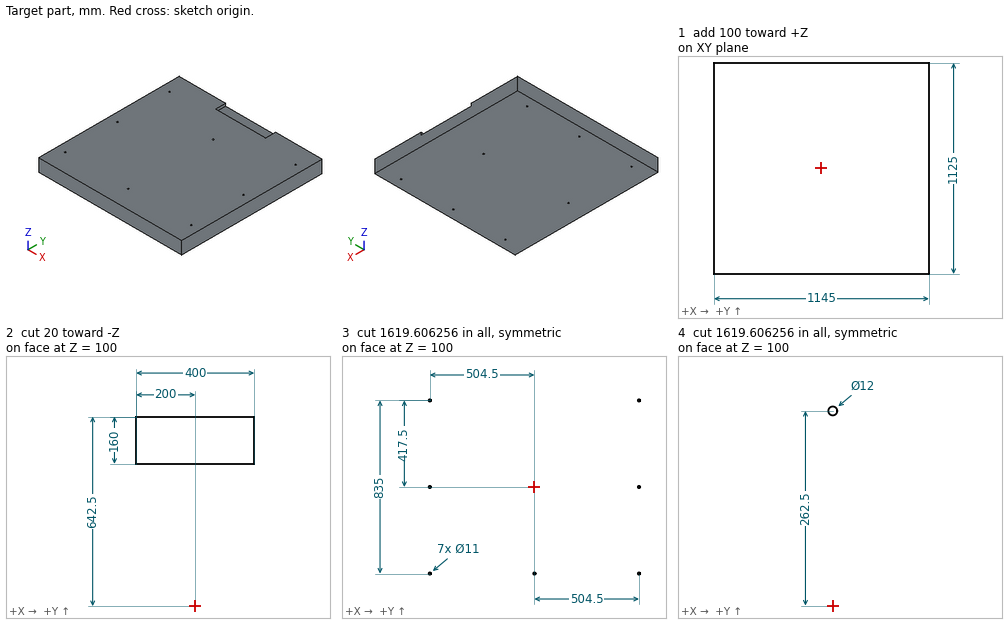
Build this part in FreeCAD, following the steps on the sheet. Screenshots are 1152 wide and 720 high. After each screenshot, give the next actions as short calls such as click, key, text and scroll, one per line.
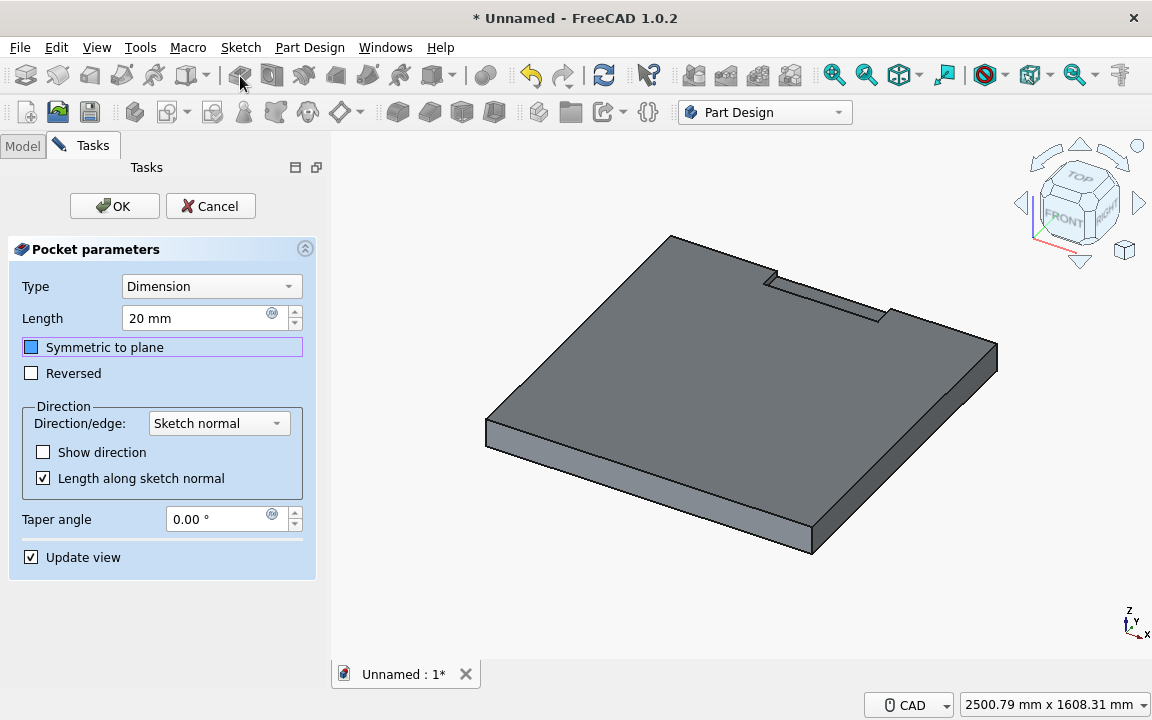
click(115, 206)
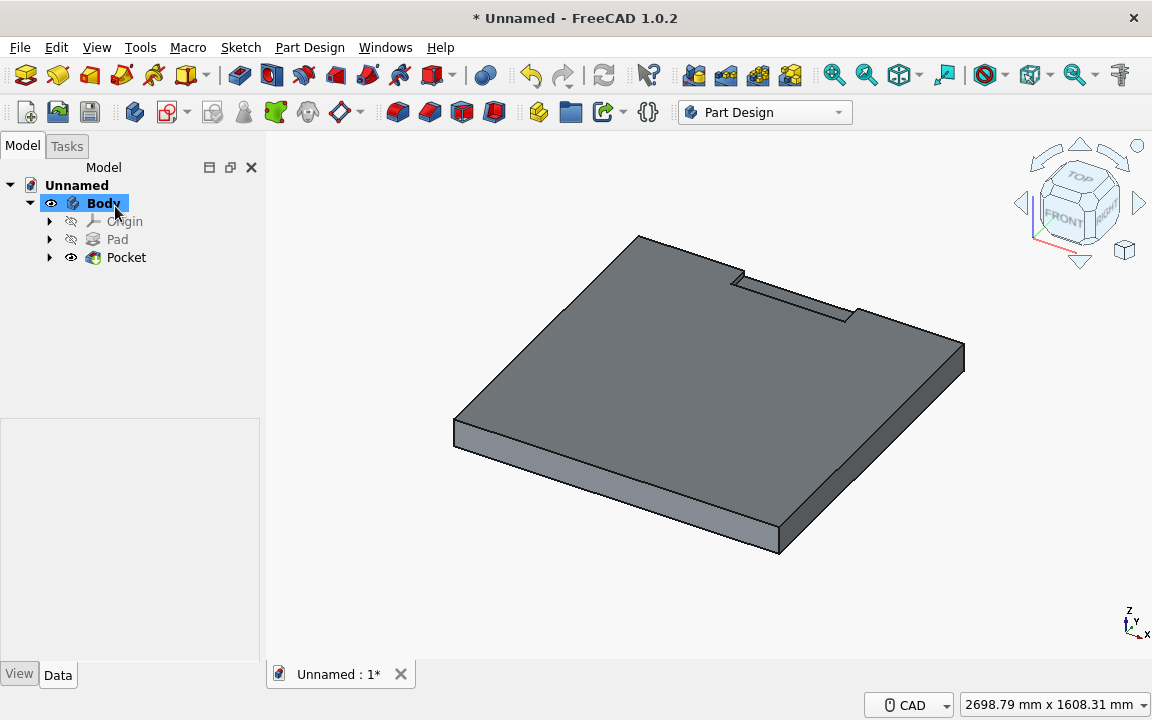
click(709, 381)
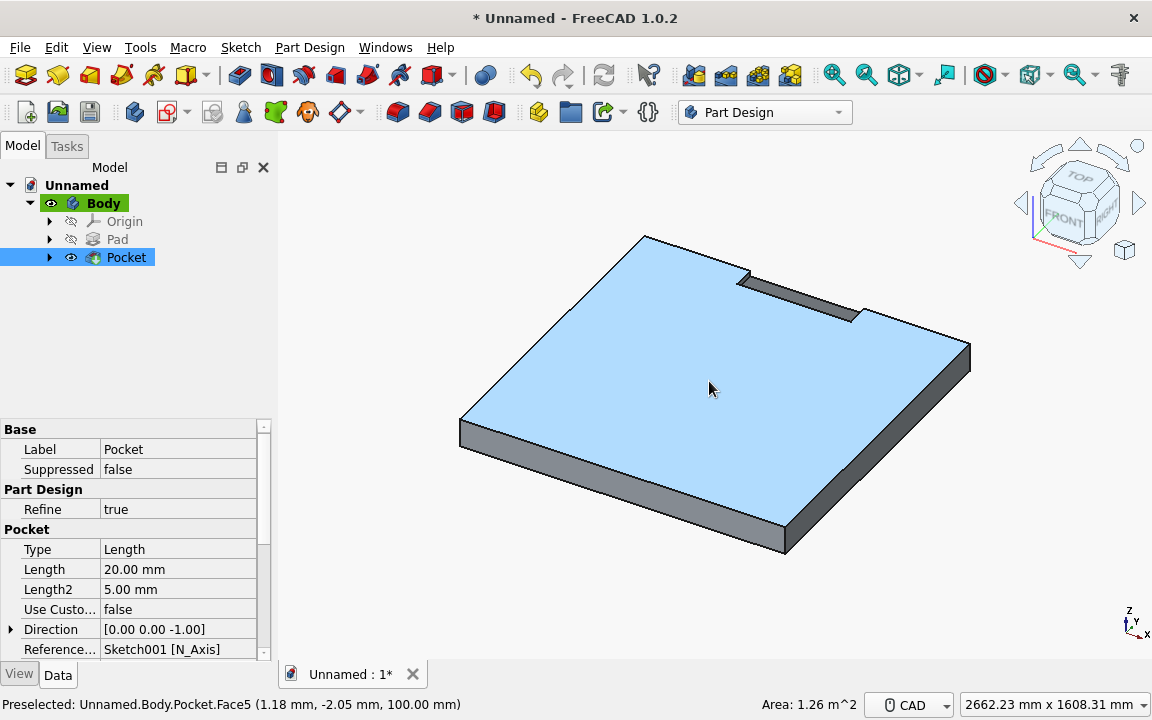
click(168, 112)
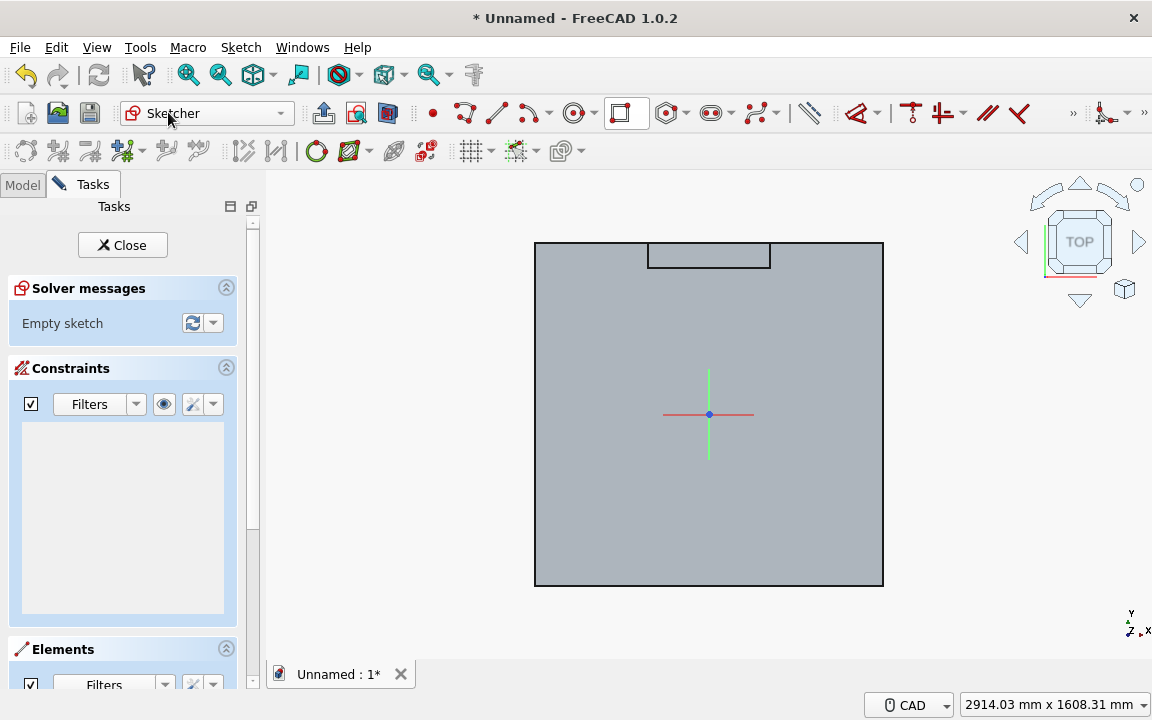
click(574, 114)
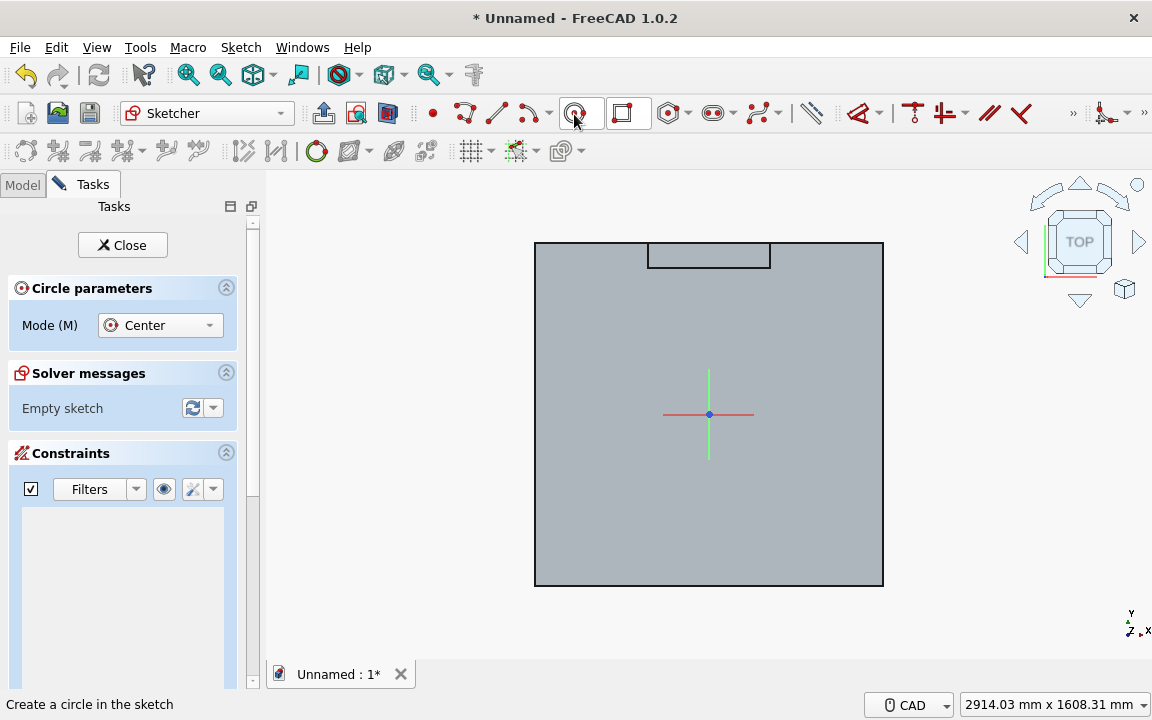
scroll(556, 288, up, 14)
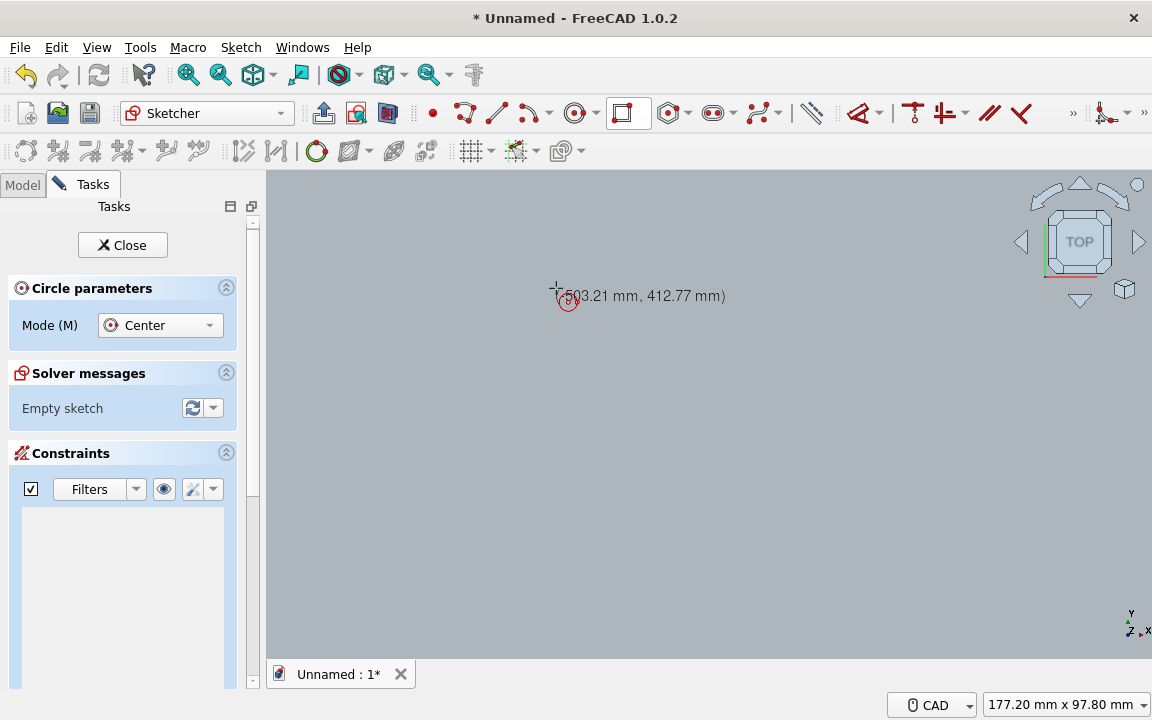
scroll(446, 258, down, 13)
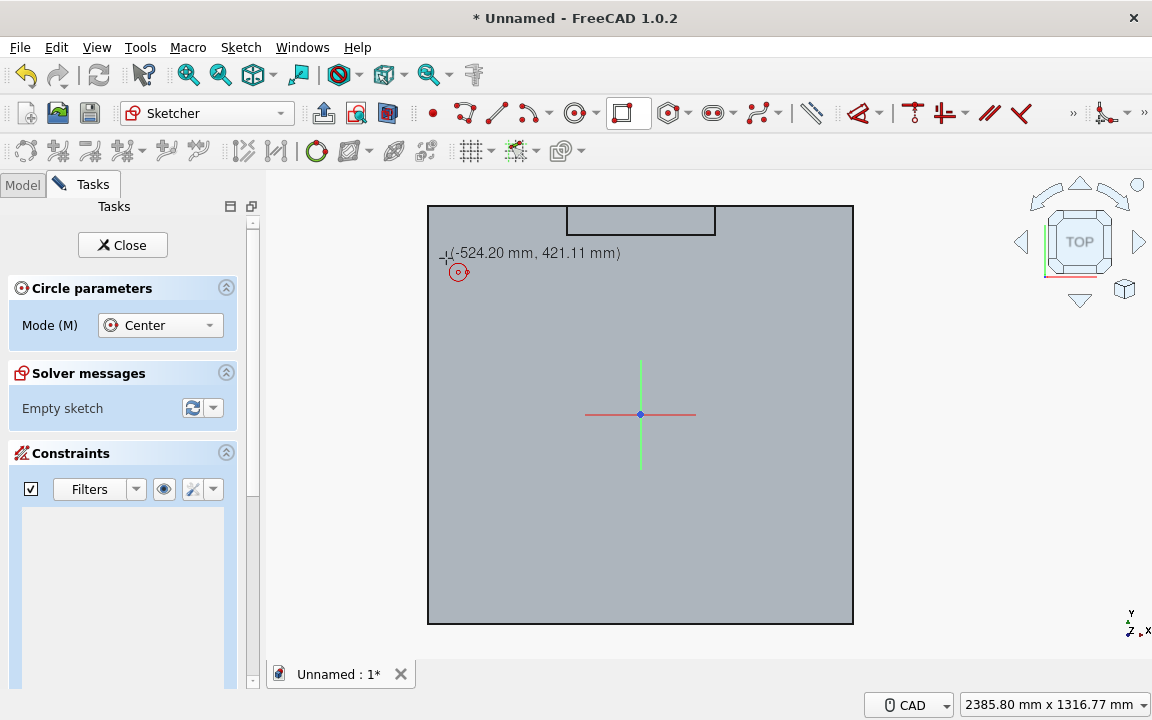
click(454, 260)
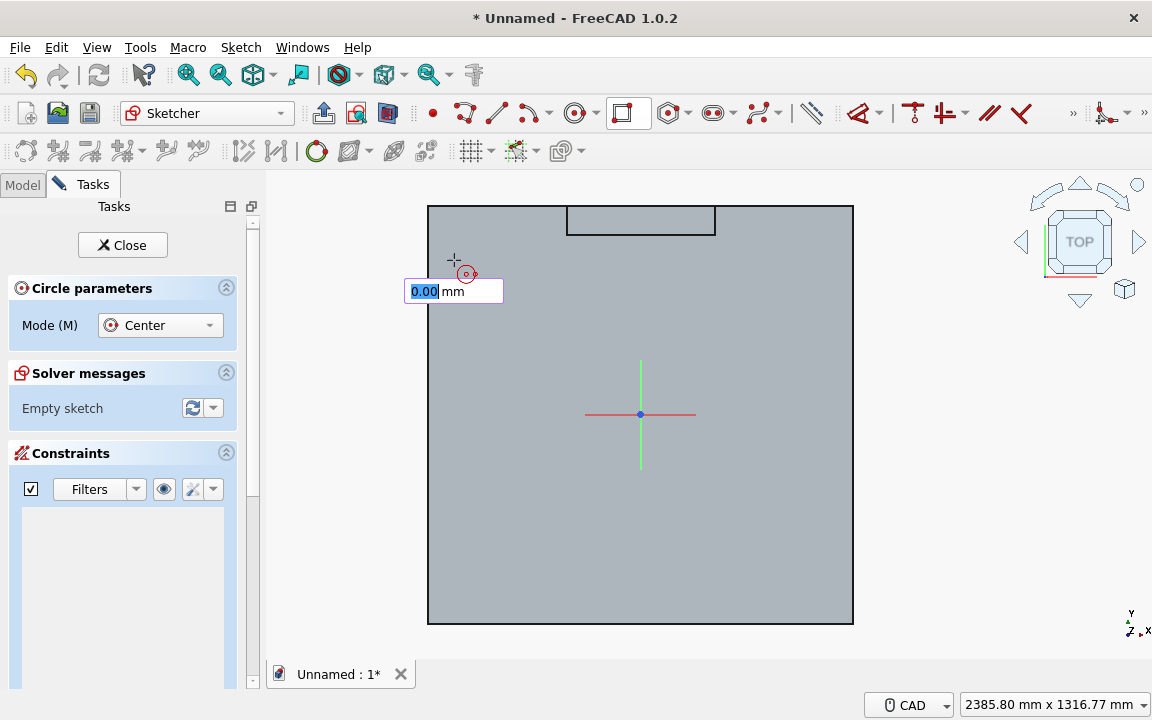
scroll(455, 258, up, 11)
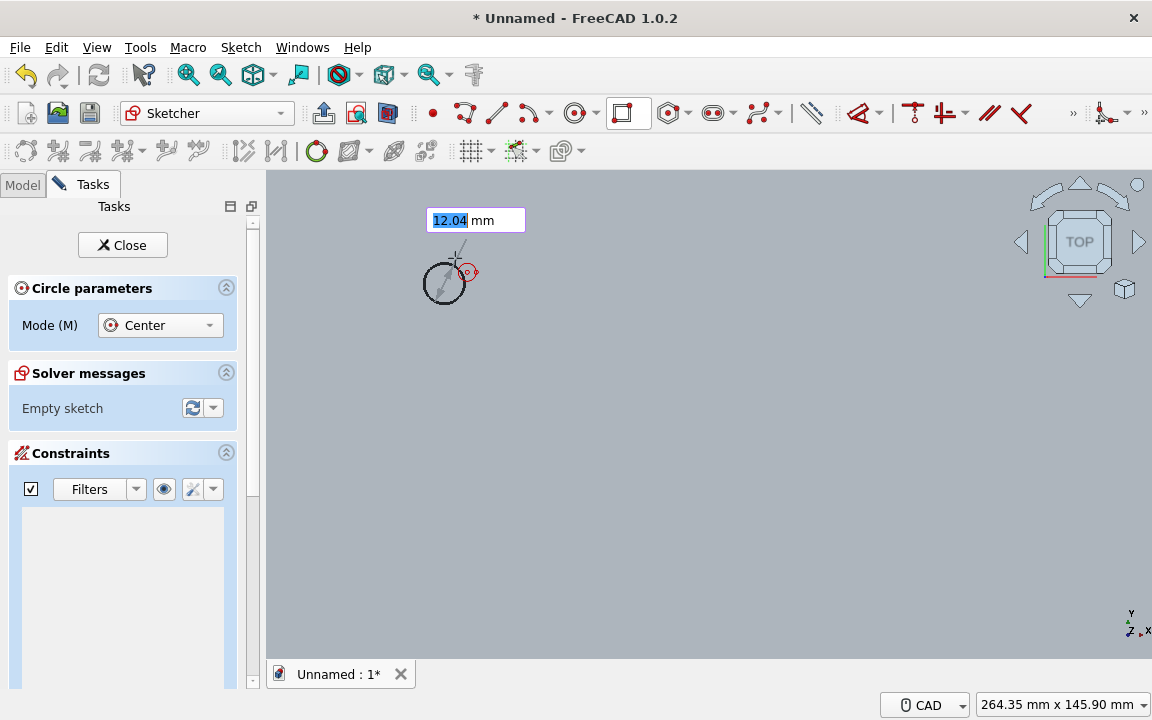
click(453, 258)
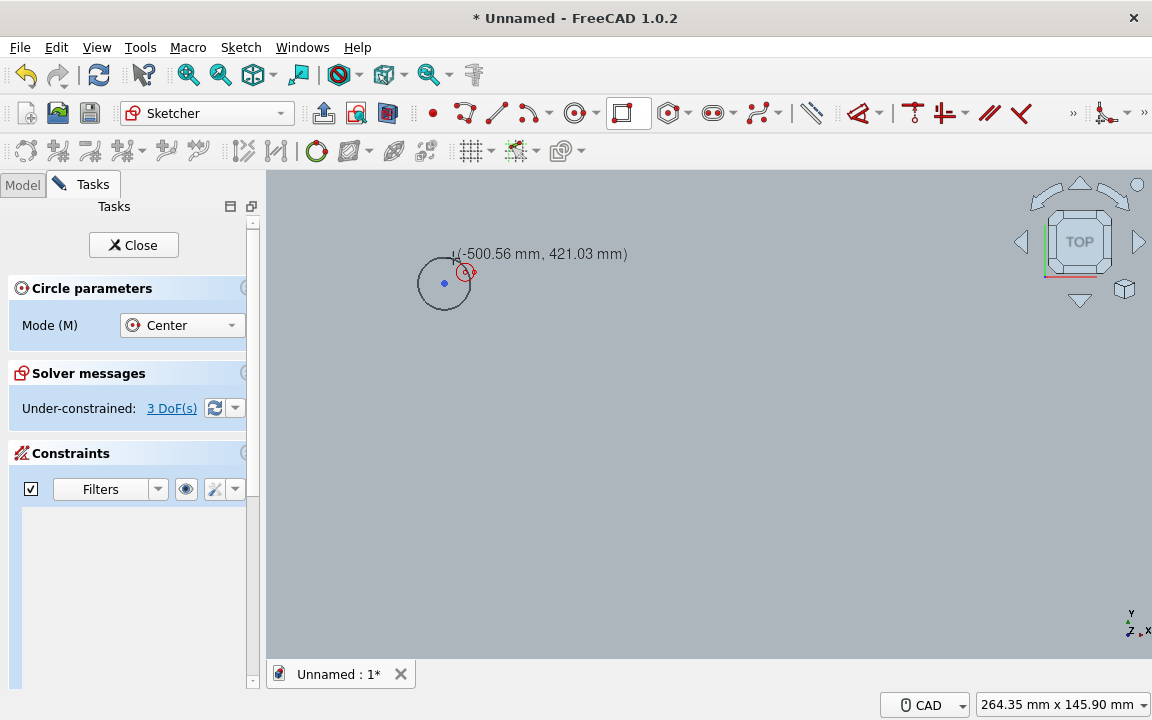
scroll(455, 258, down, 11)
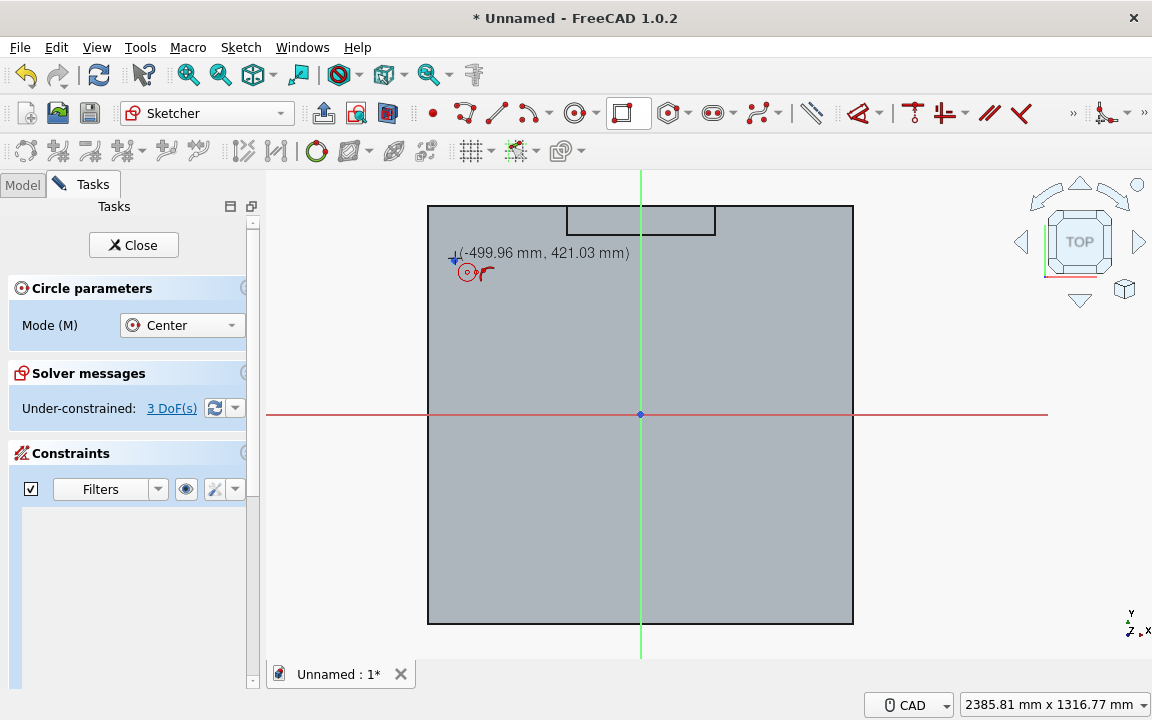
scroll(454, 570, up, 13)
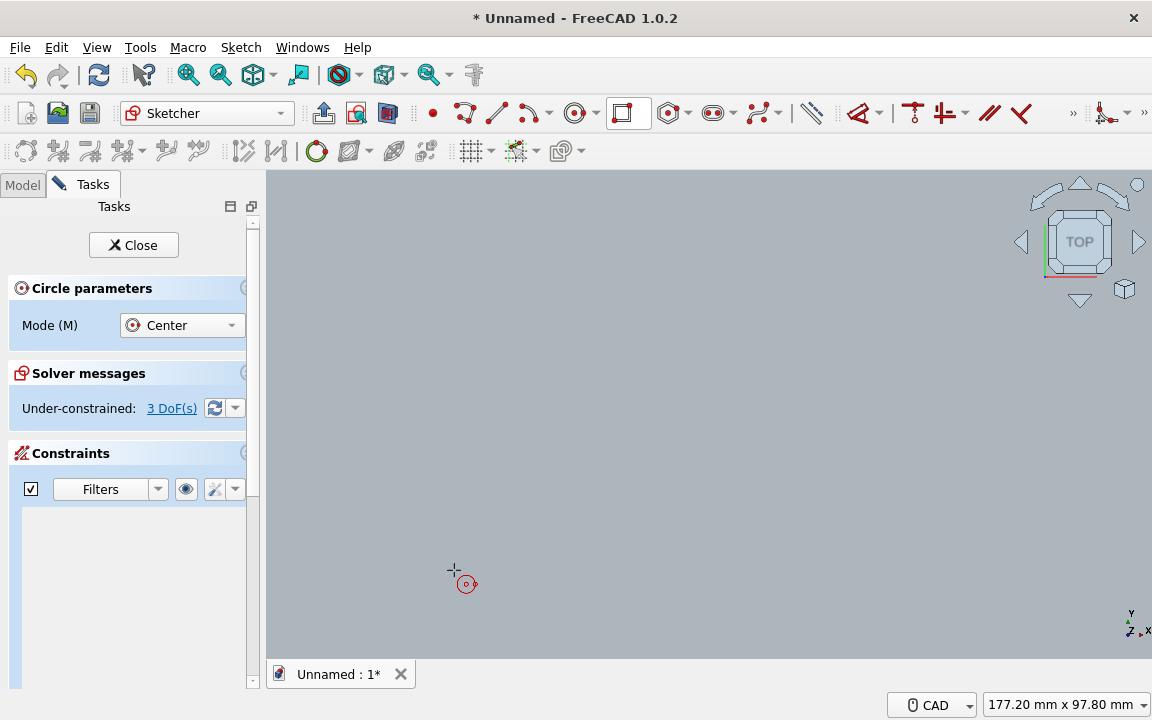
scroll(454, 571, down, 13)